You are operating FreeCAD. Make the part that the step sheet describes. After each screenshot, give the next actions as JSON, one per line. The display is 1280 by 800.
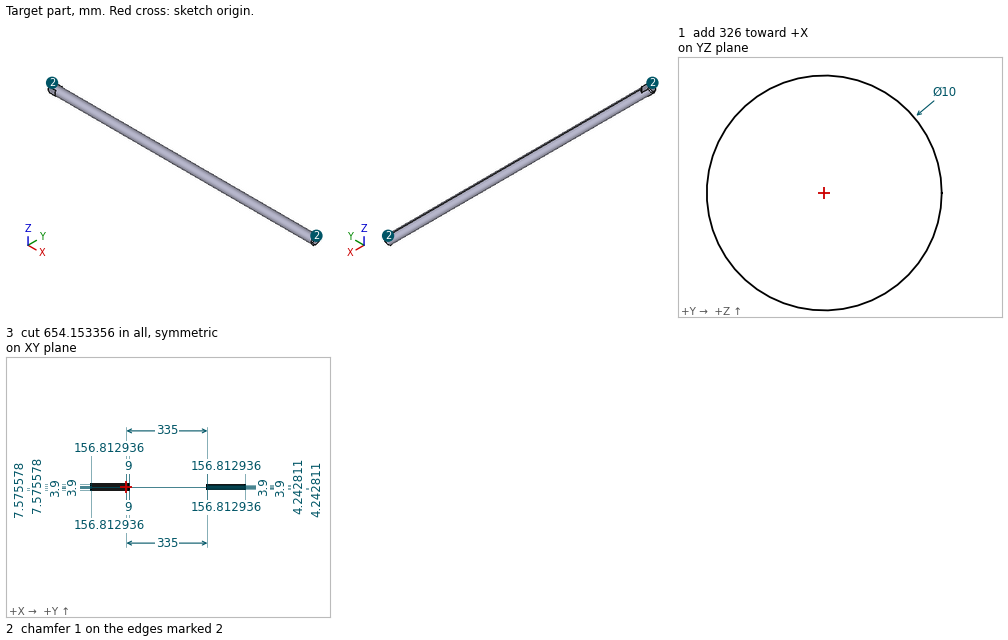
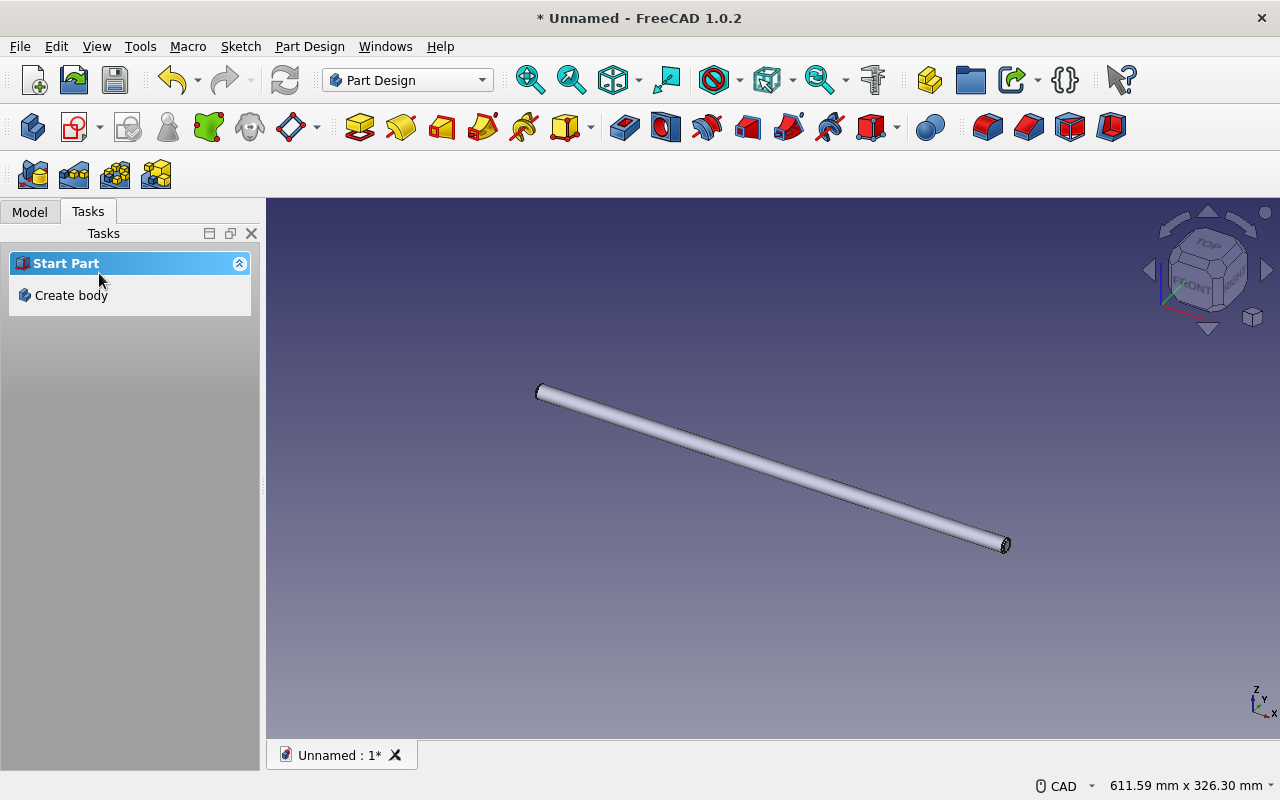
{"action": "left_click", "coordinate": [74, 128]}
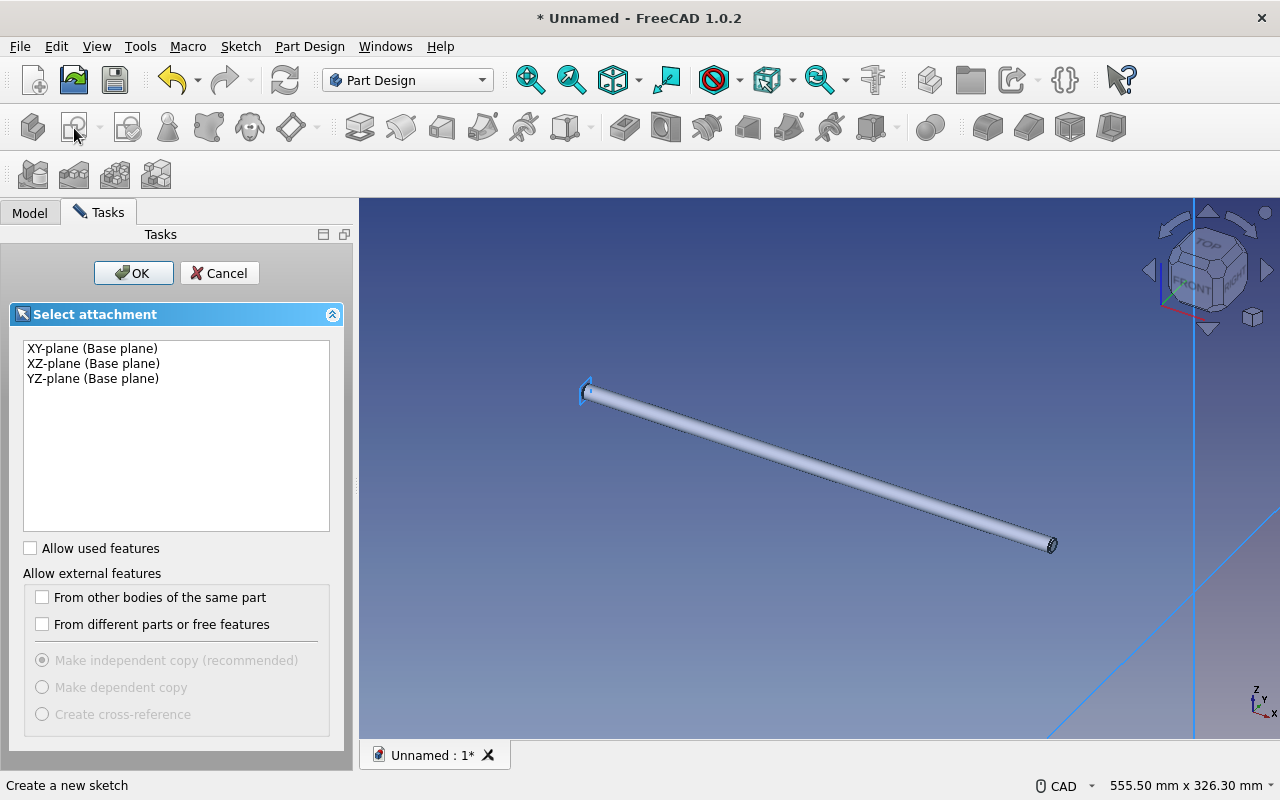
{"action": "left_click", "coordinate": [84, 348]}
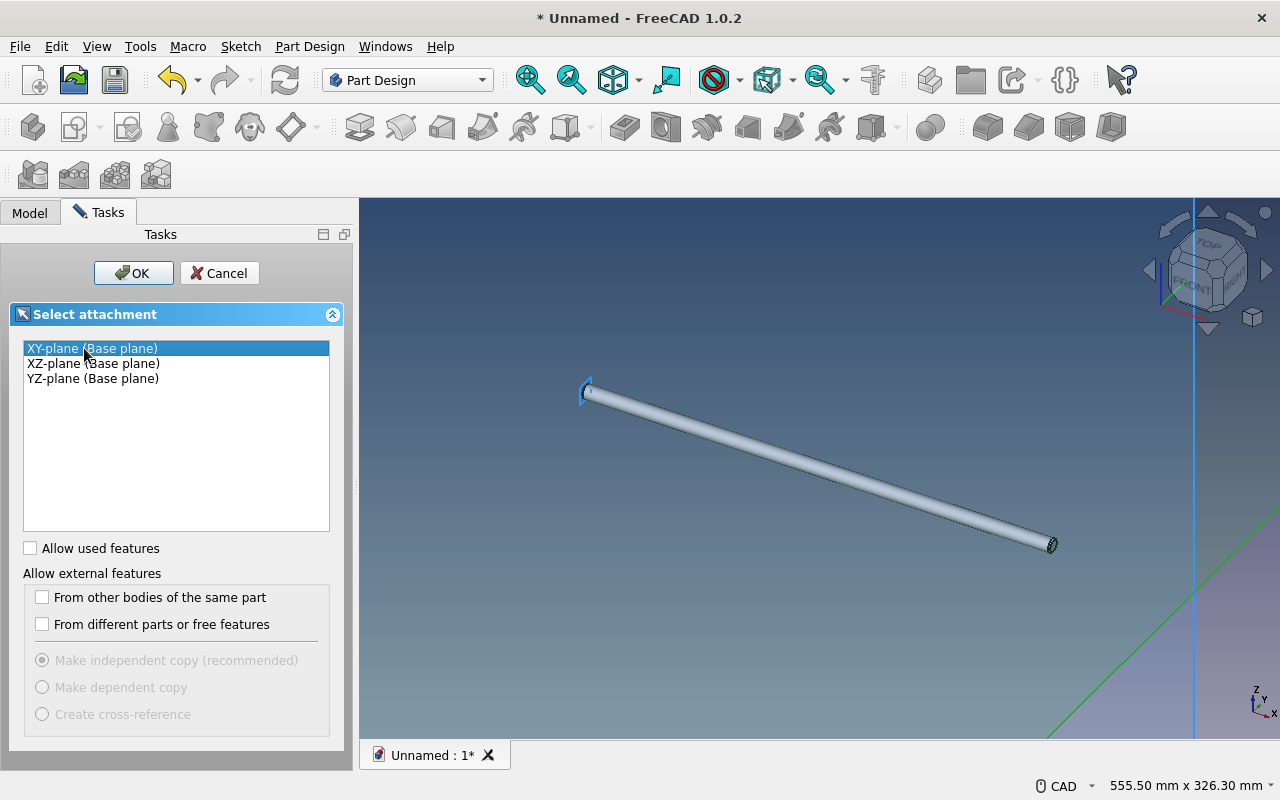
{"action": "left_click", "coordinate": [134, 273]}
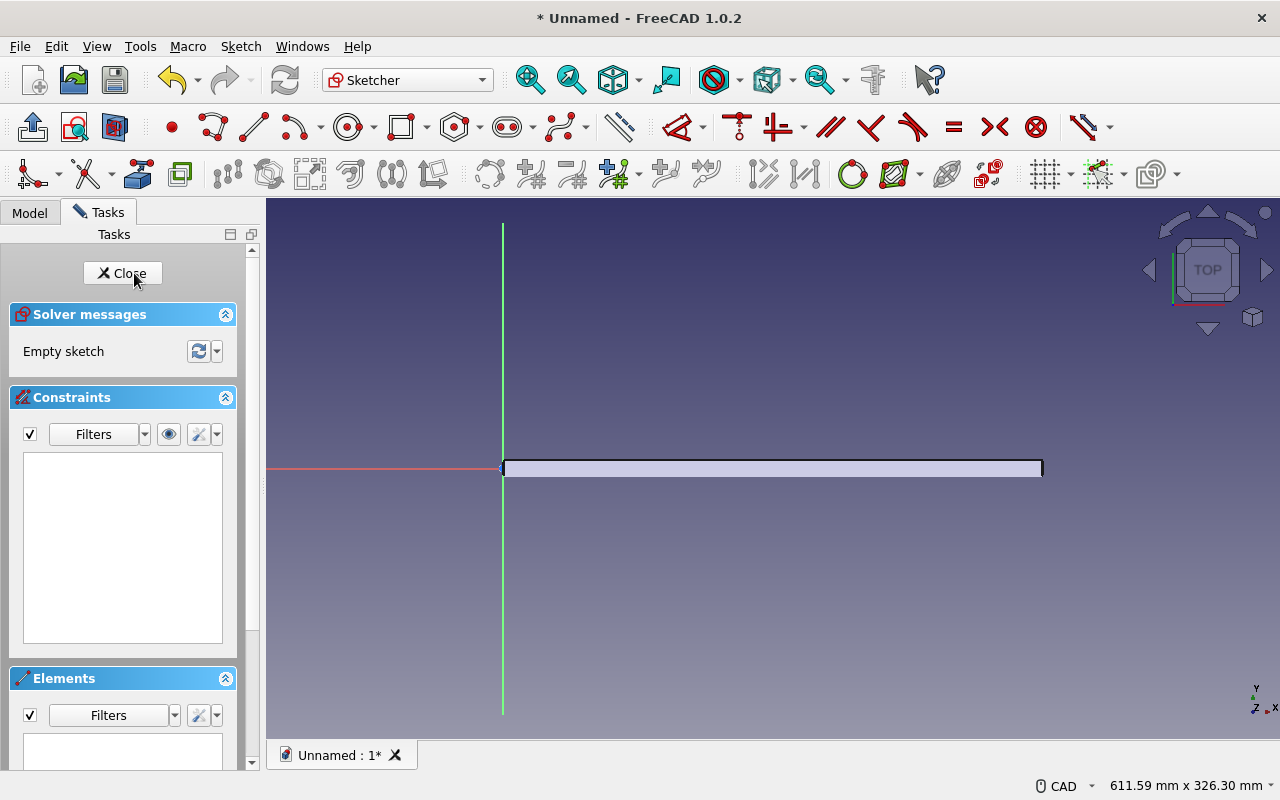
{"action": "left_click", "coordinate": [115, 128]}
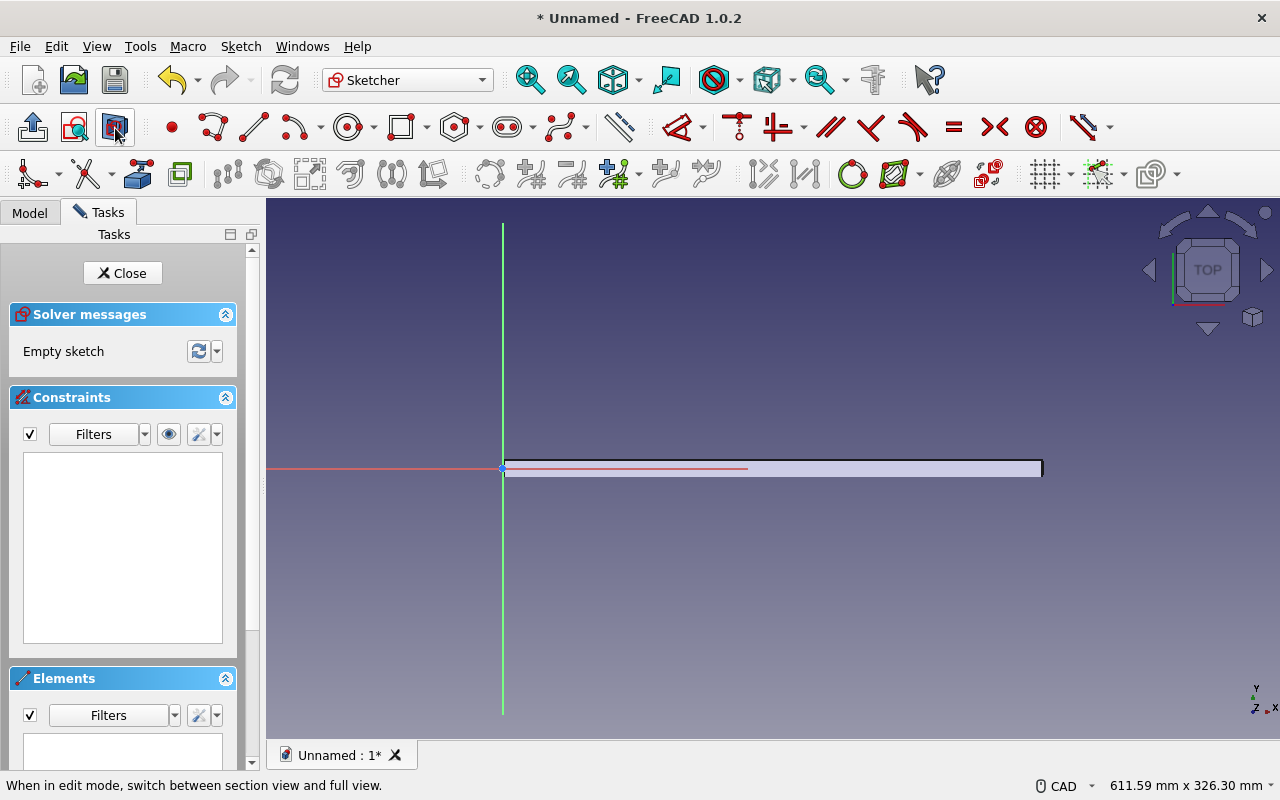
{"action": "scroll", "coordinate": [603, 468], "scroll_direction": "down", "scroll_amount": 3}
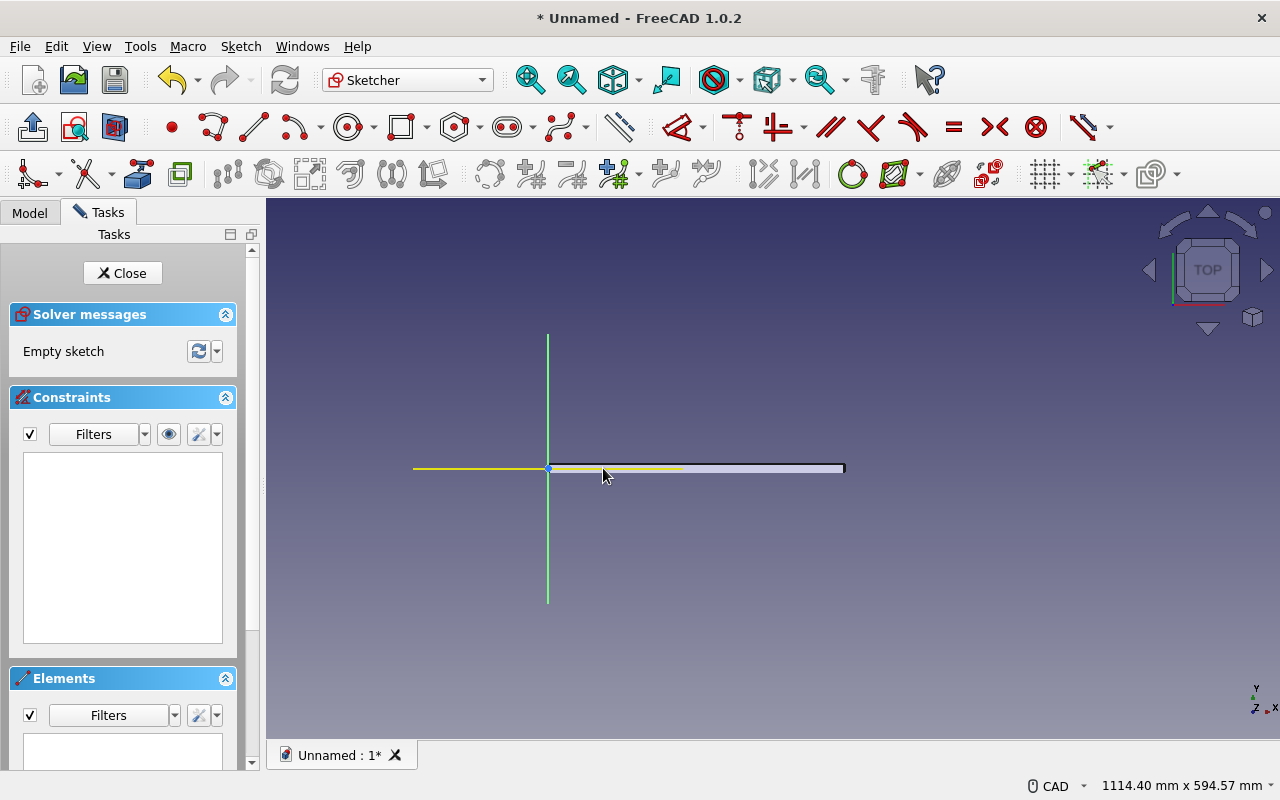
{"action": "left_click", "coordinate": [400, 128]}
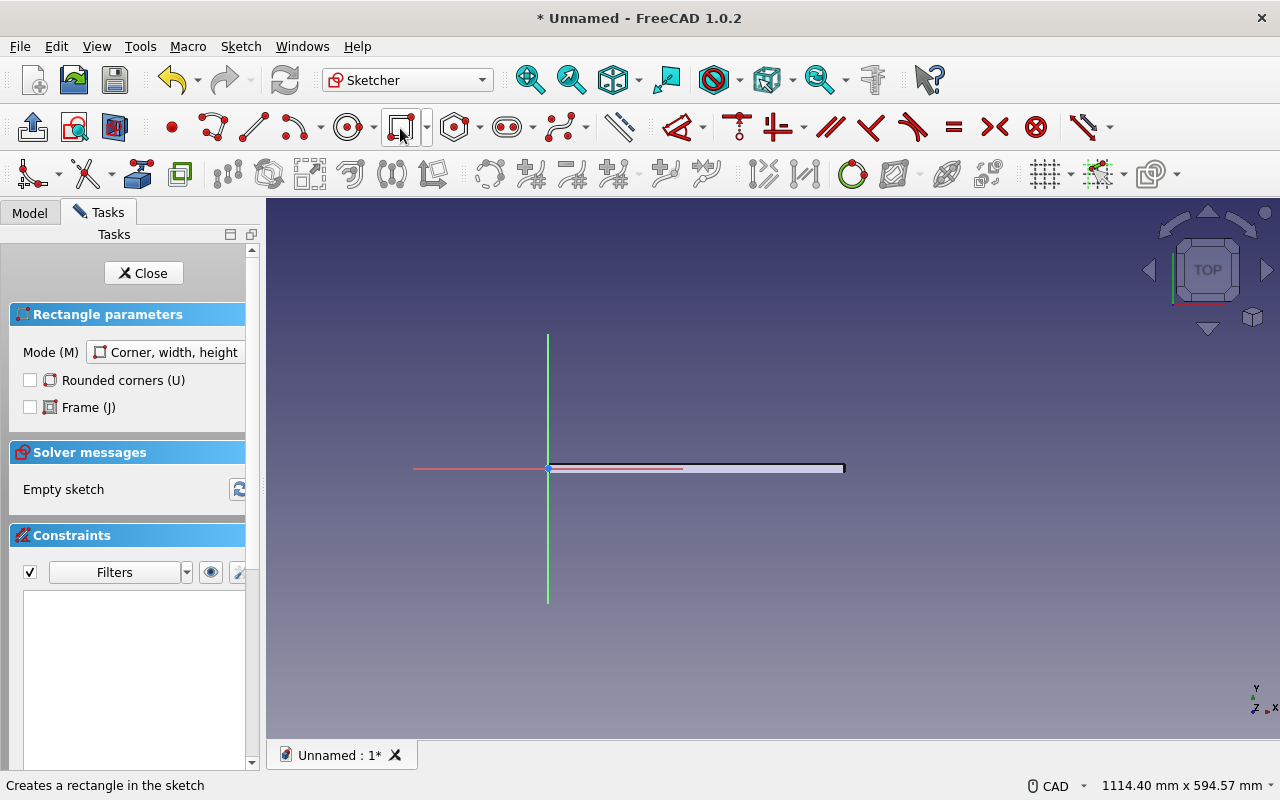
{"action": "scroll", "coordinate": [853, 461], "scroll_direction": "up", "scroll_amount": 8}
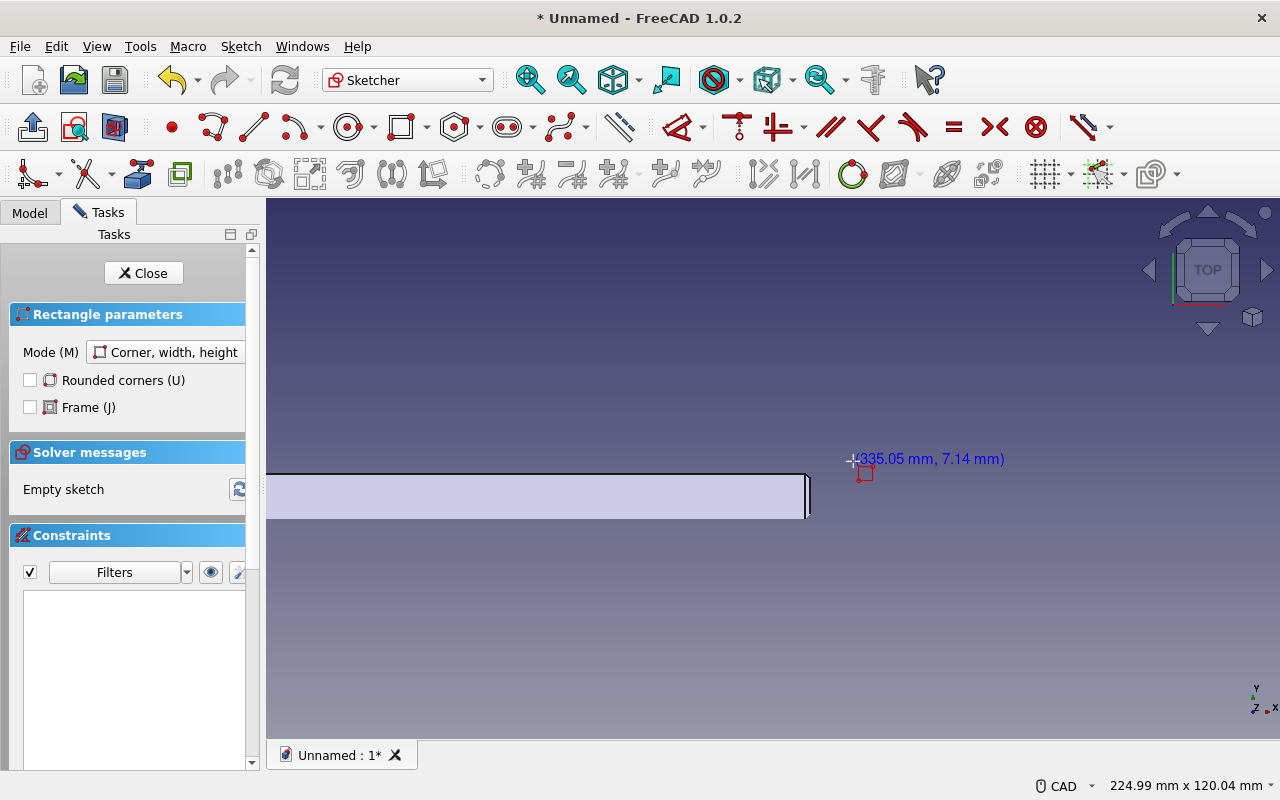
{"action": "left_click", "coordinate": [850, 460]}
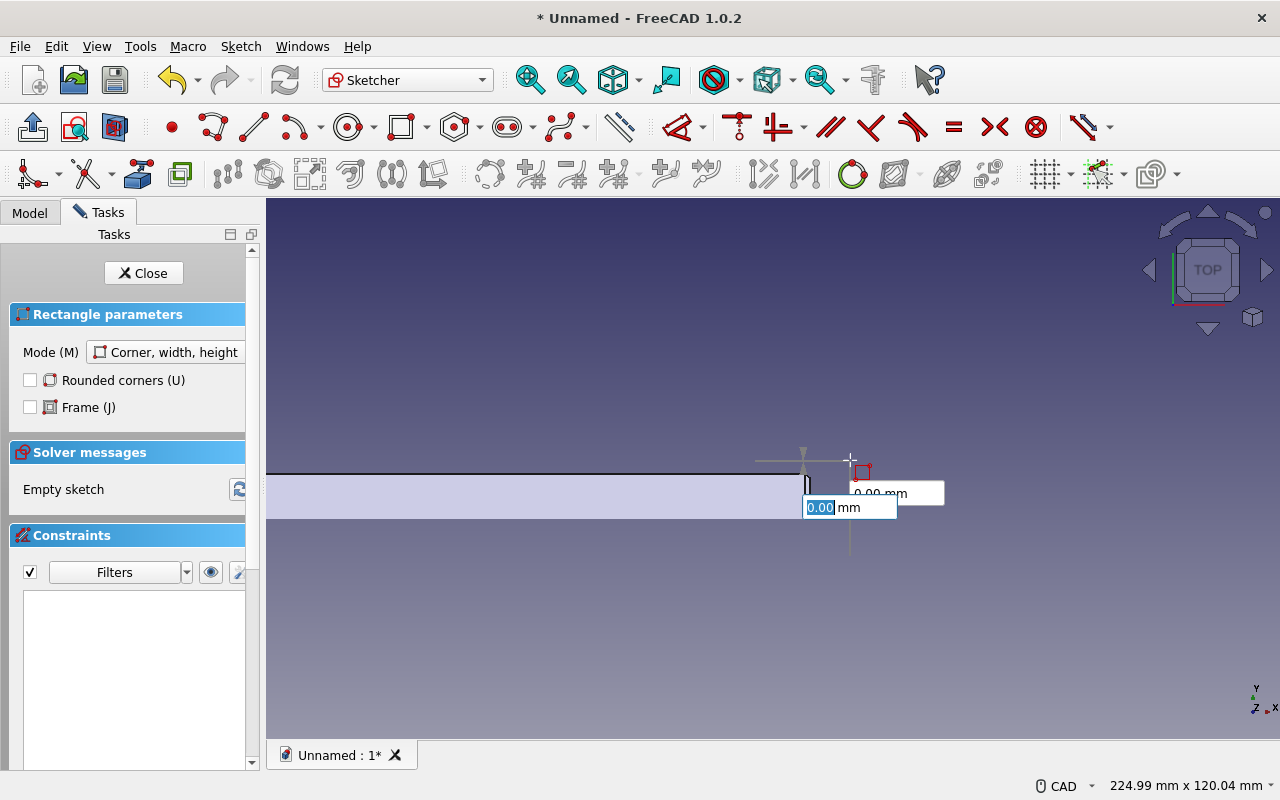
{"action": "scroll", "coordinate": [853, 461], "scroll_direction": "down", "scroll_amount": 8}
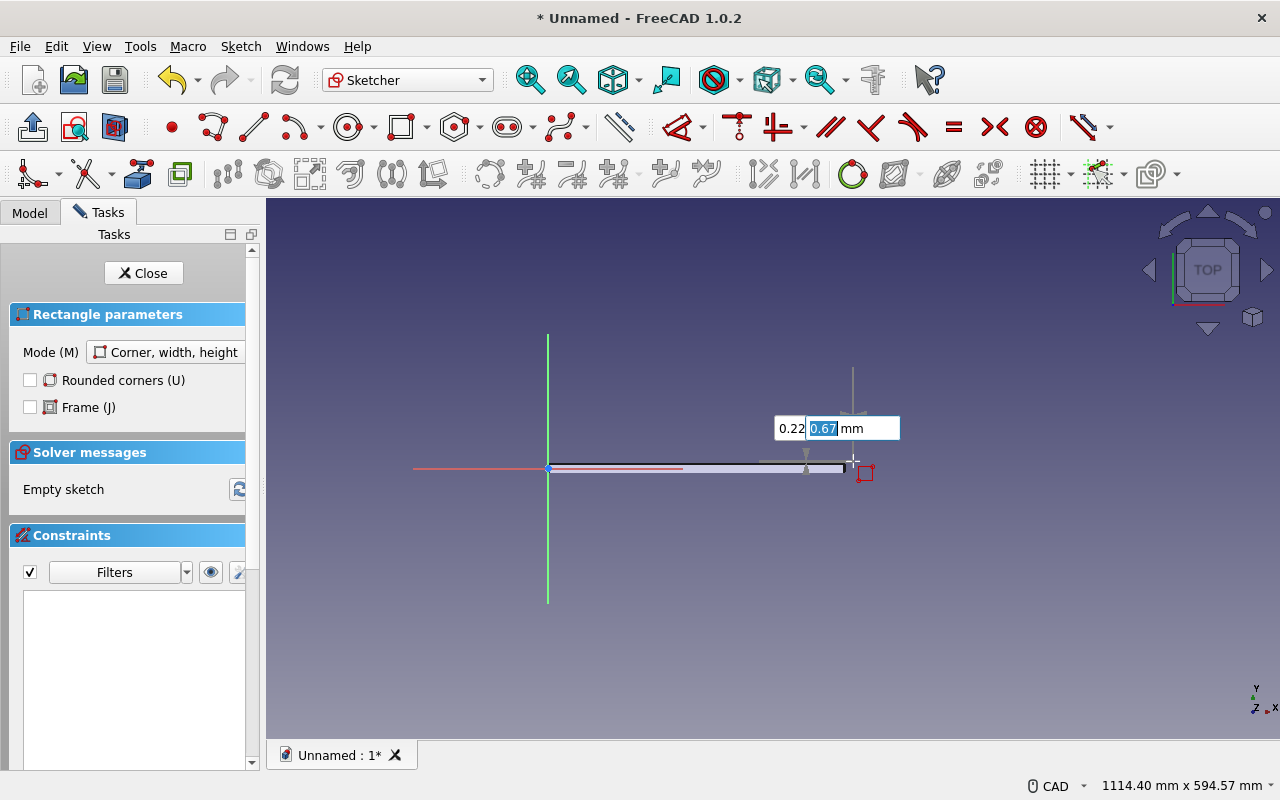
{"action": "scroll", "coordinate": [996, 465], "scroll_direction": "up", "scroll_amount": 8}